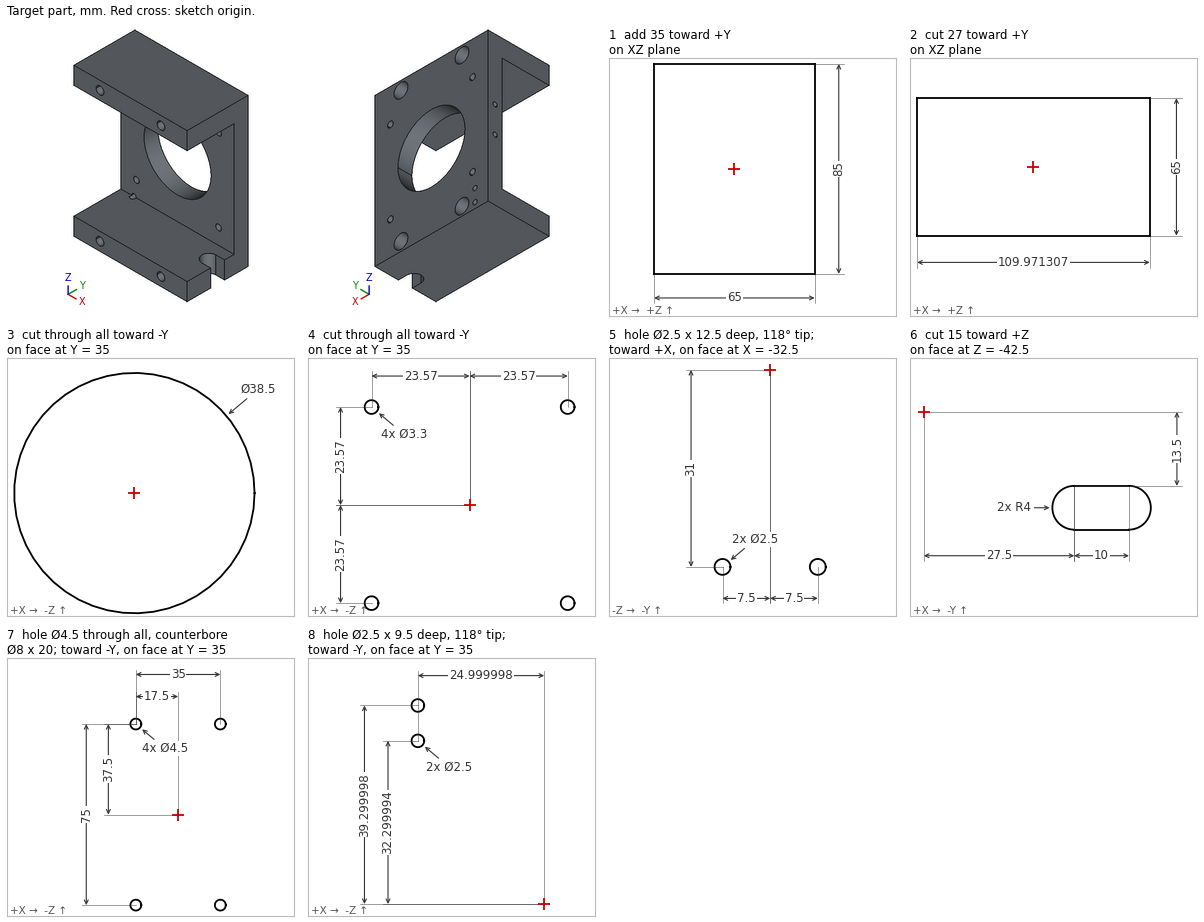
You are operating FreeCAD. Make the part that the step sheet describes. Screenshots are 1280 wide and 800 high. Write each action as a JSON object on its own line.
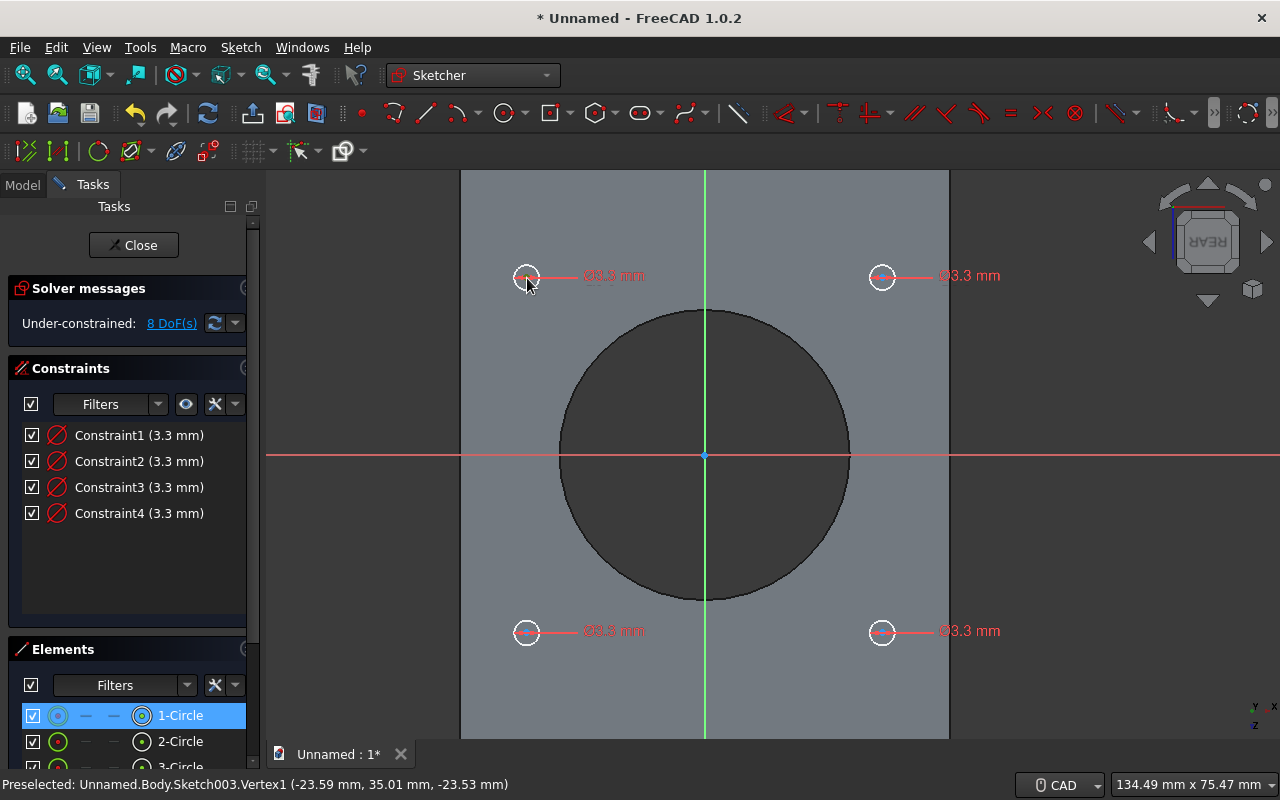
{"action": "left_click", "coordinate": [882, 278]}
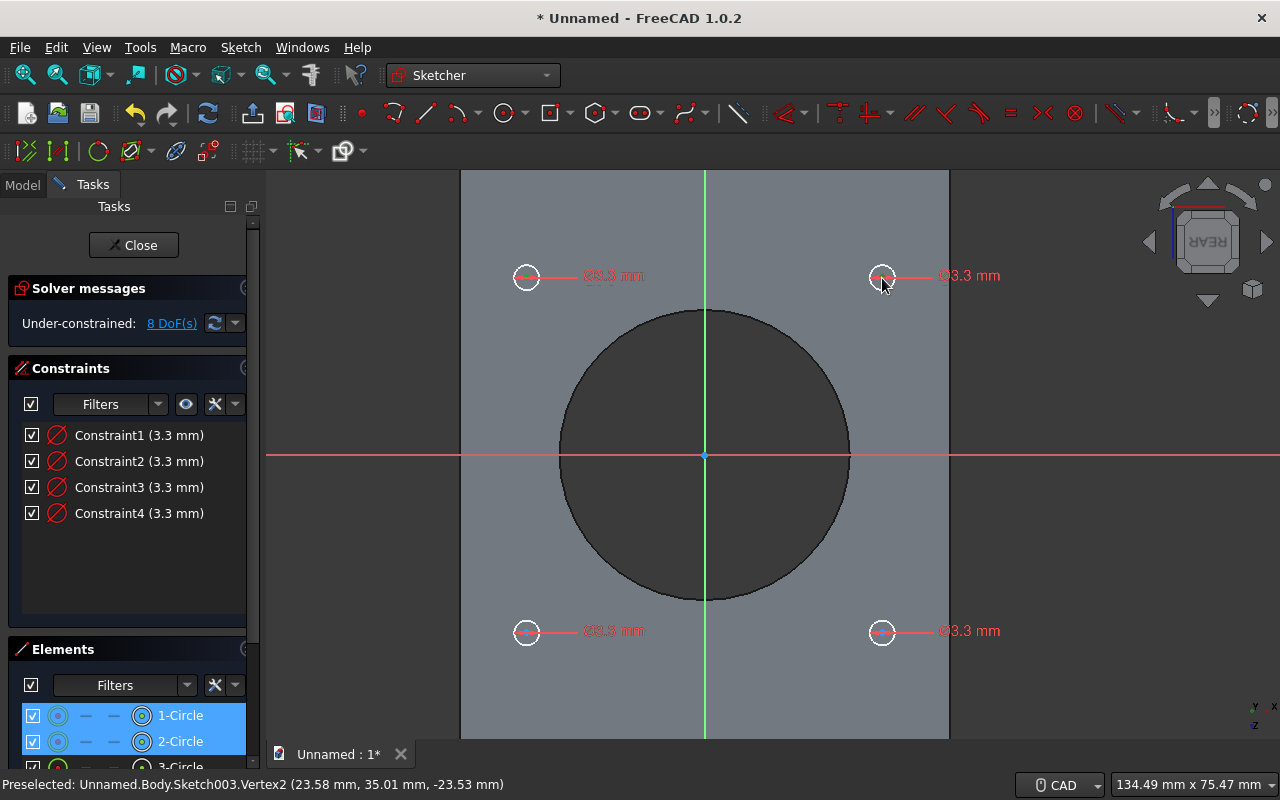
{"action": "left_click", "coordinate": [892, 114]}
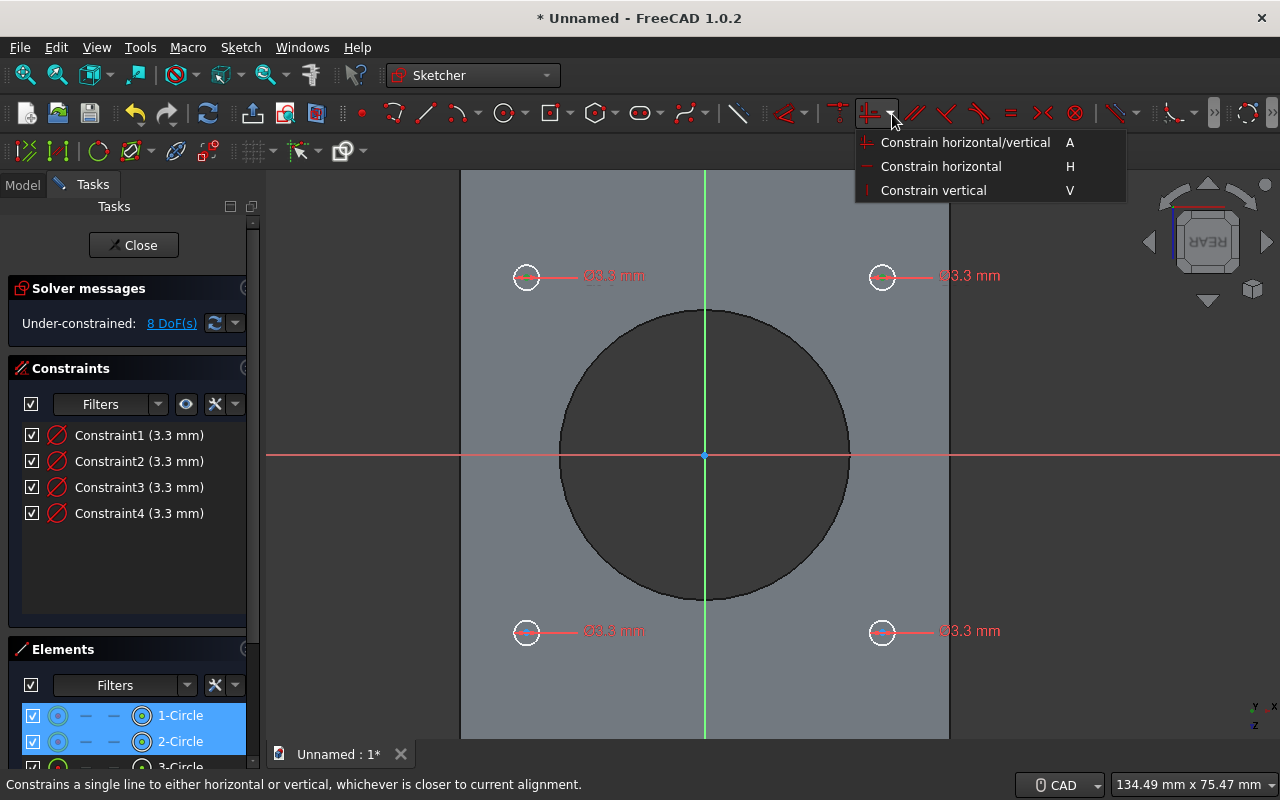
{"action": "left_click", "coordinate": [991, 166]}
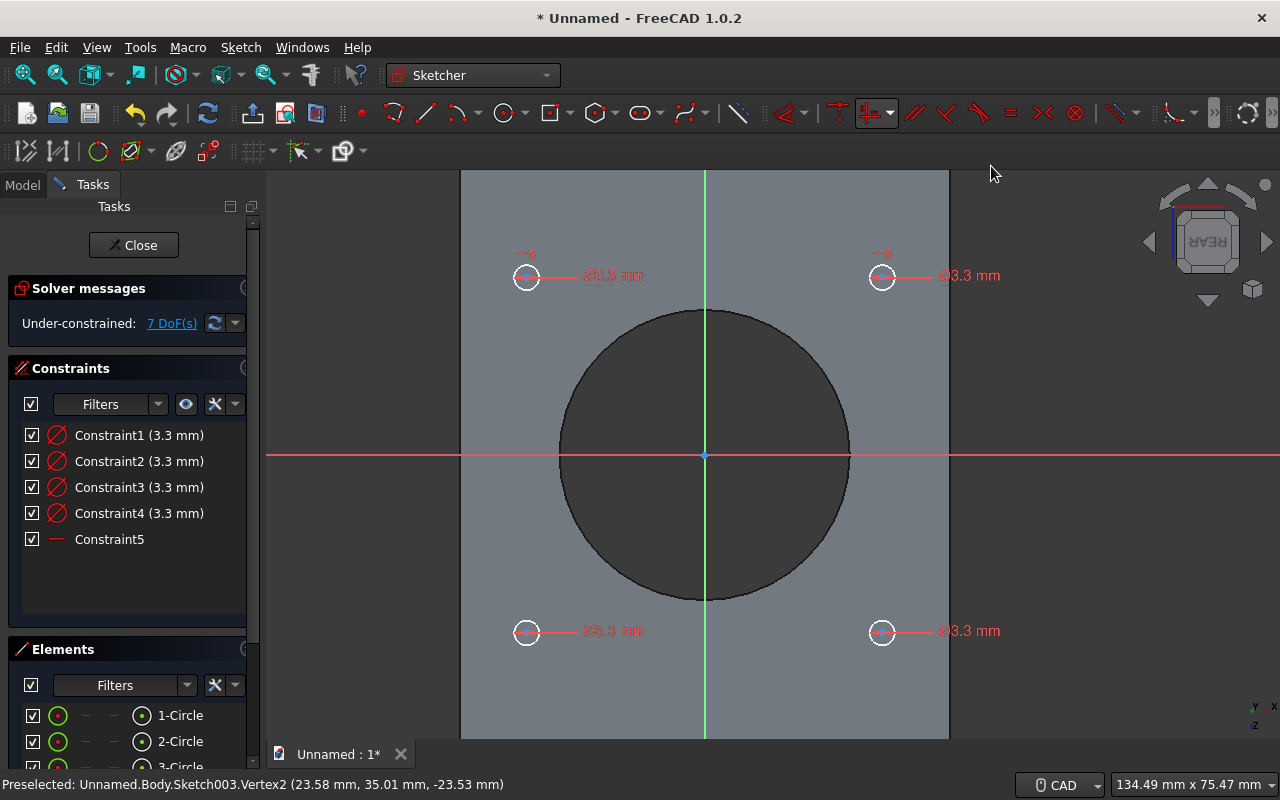
{"action": "left_click", "coordinate": [527, 278]}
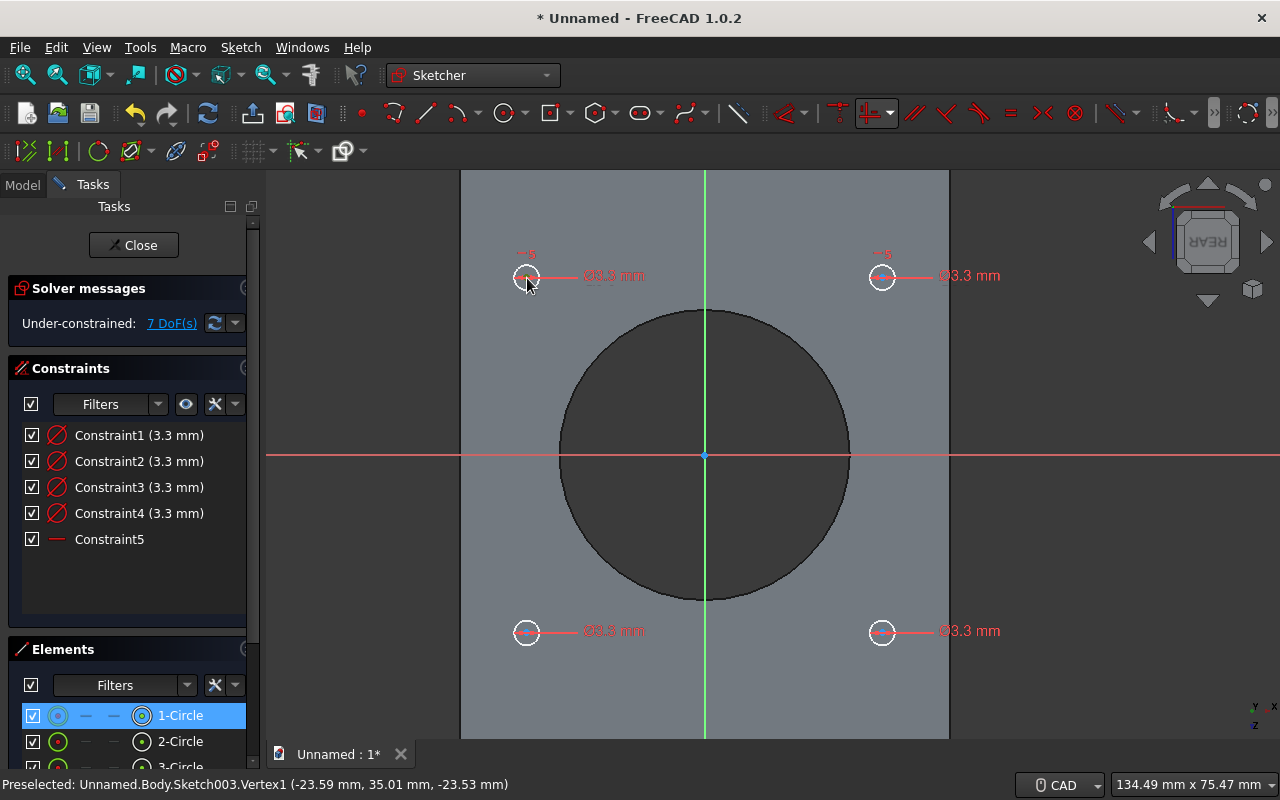
{"action": "left_click", "coordinate": [527, 633]}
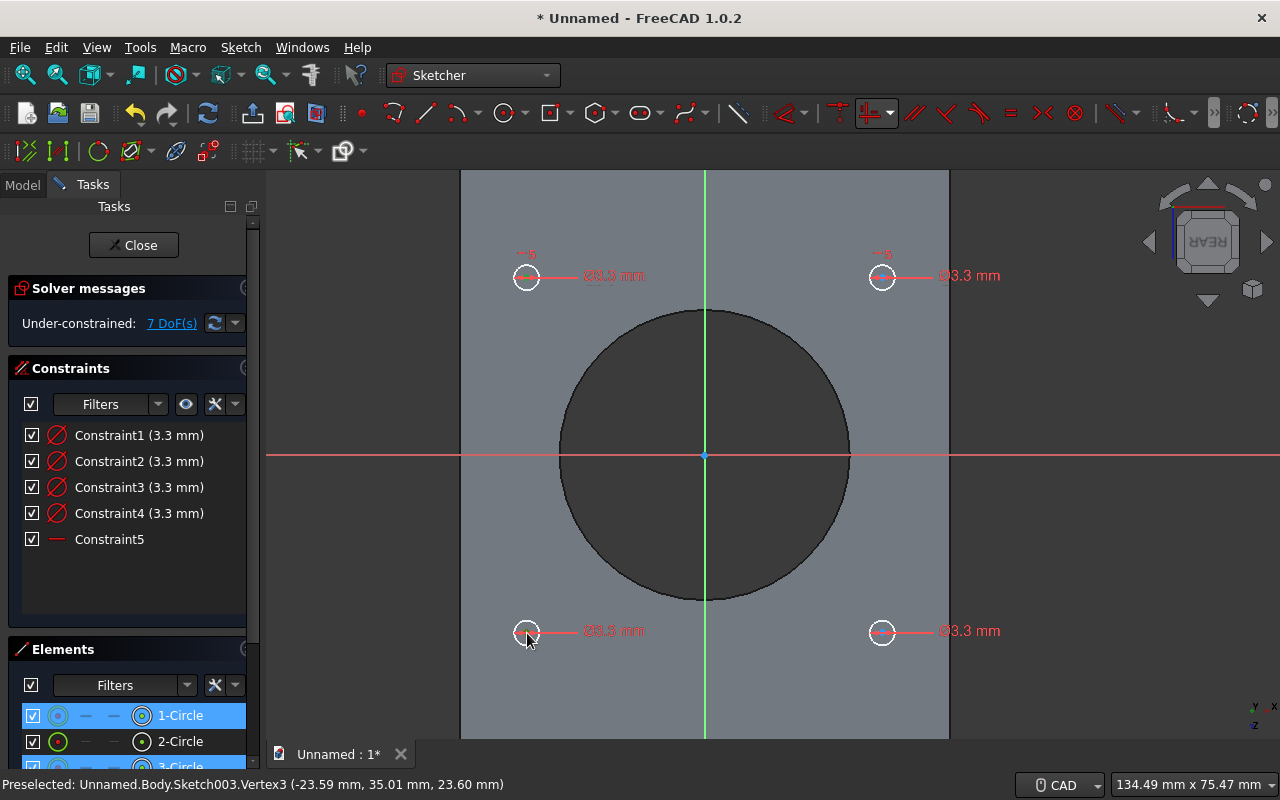
{"action": "left_click", "coordinate": [892, 114]}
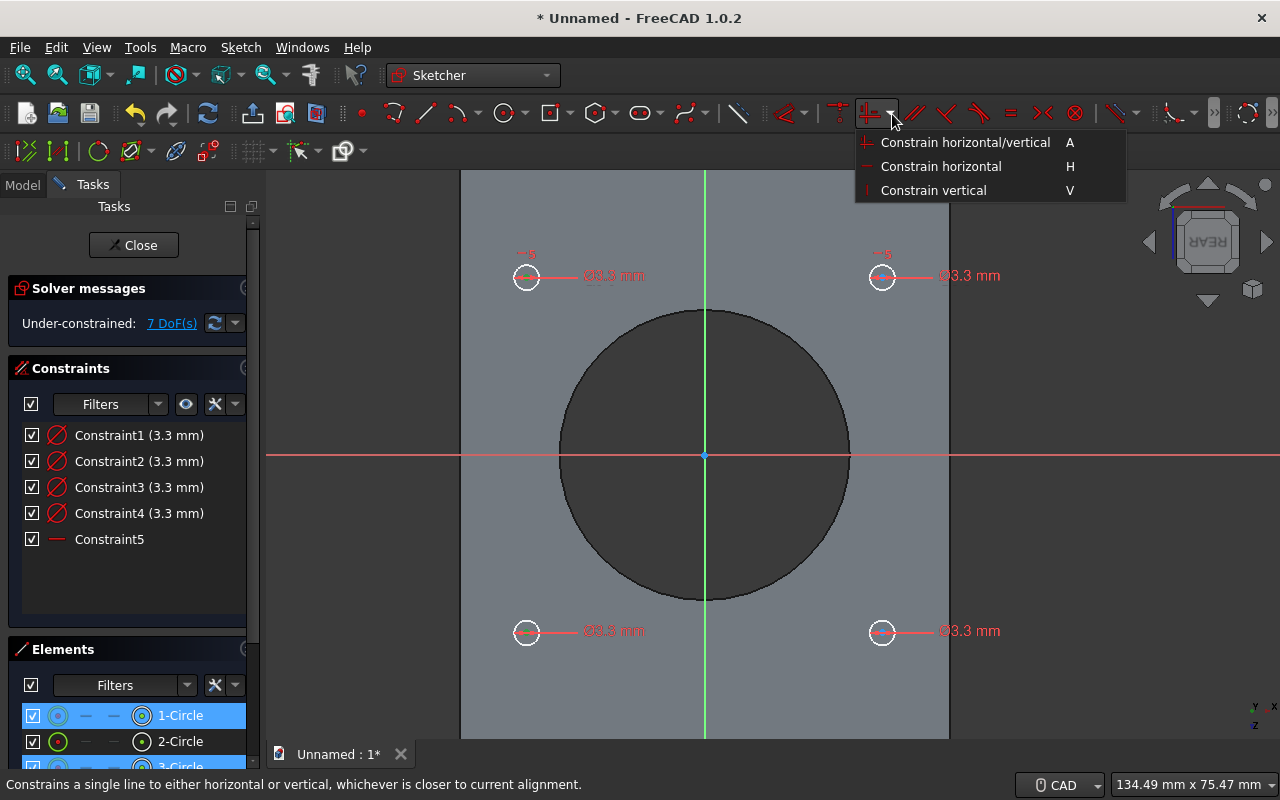
{"action": "left_click", "coordinate": [991, 190]}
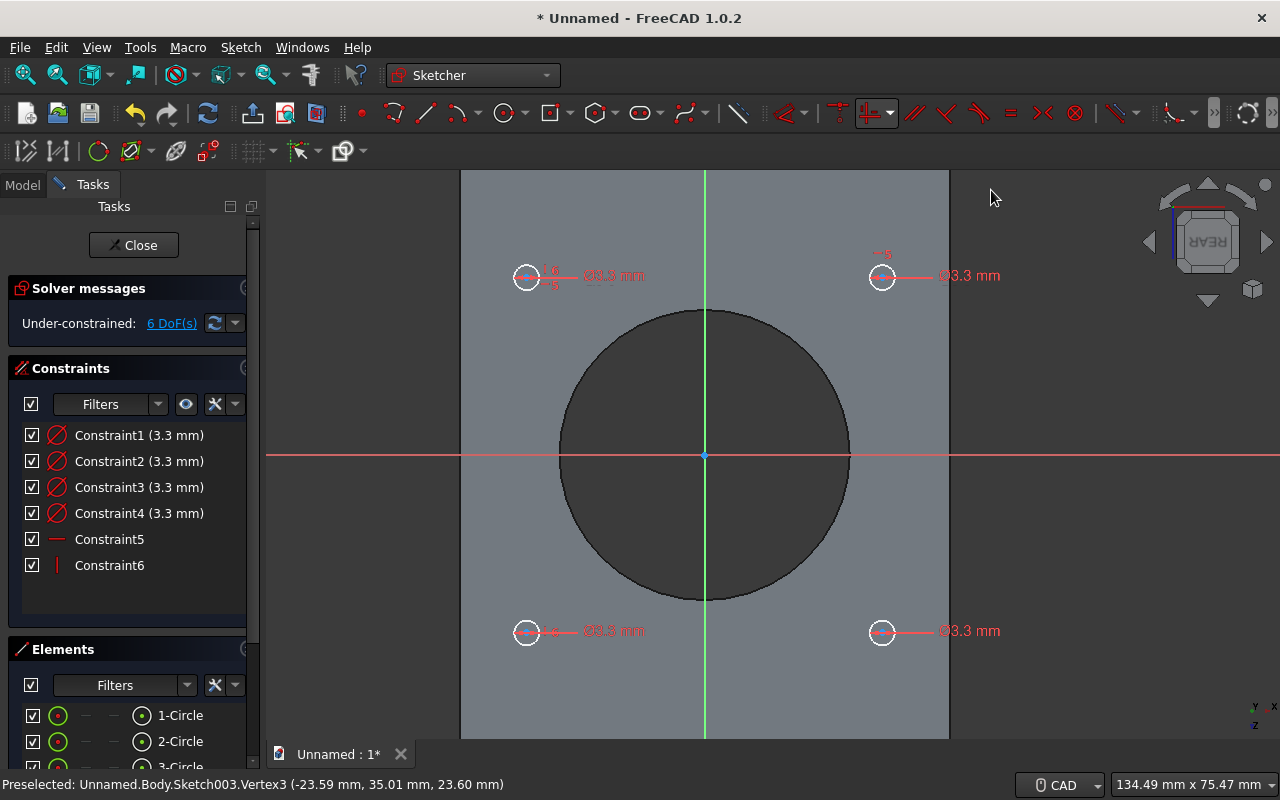
{"action": "left_click", "coordinate": [882, 278]}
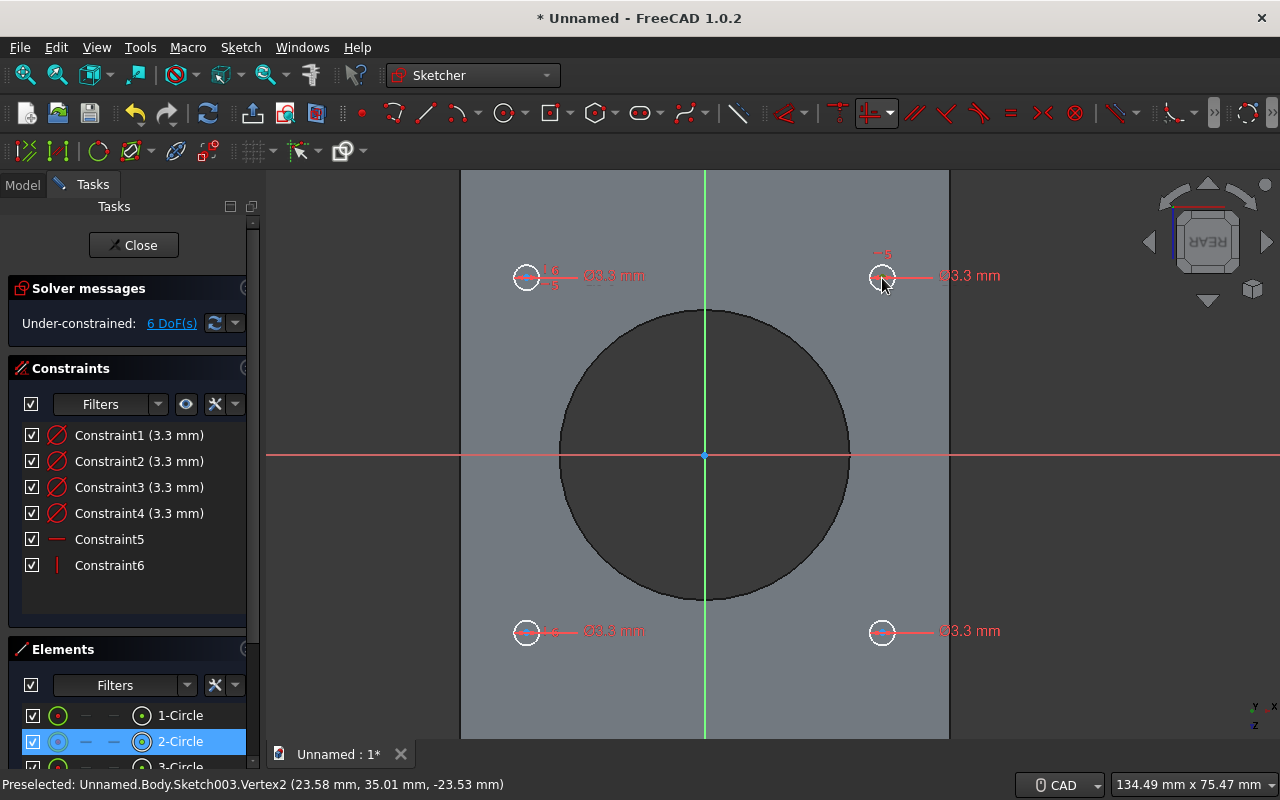
{"action": "left_click", "coordinate": [882, 633]}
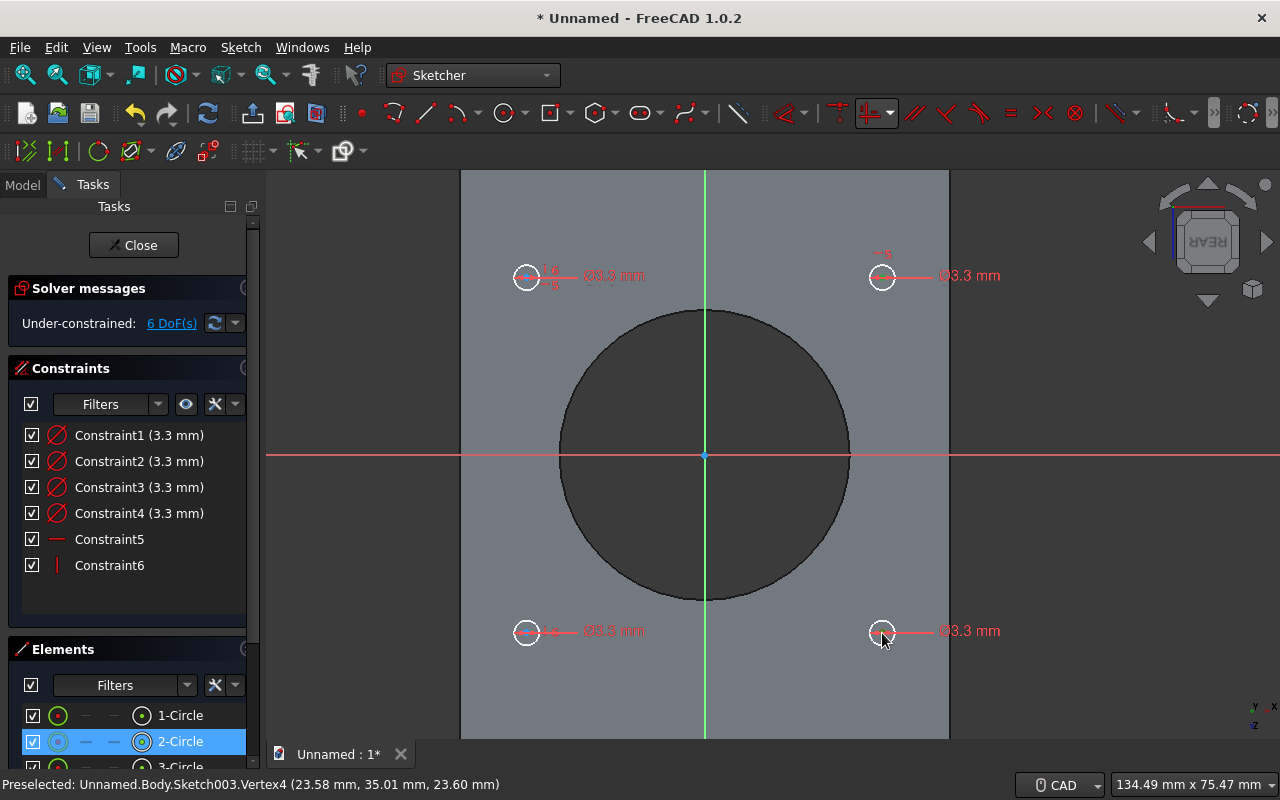
{"action": "key", "text": "v"}